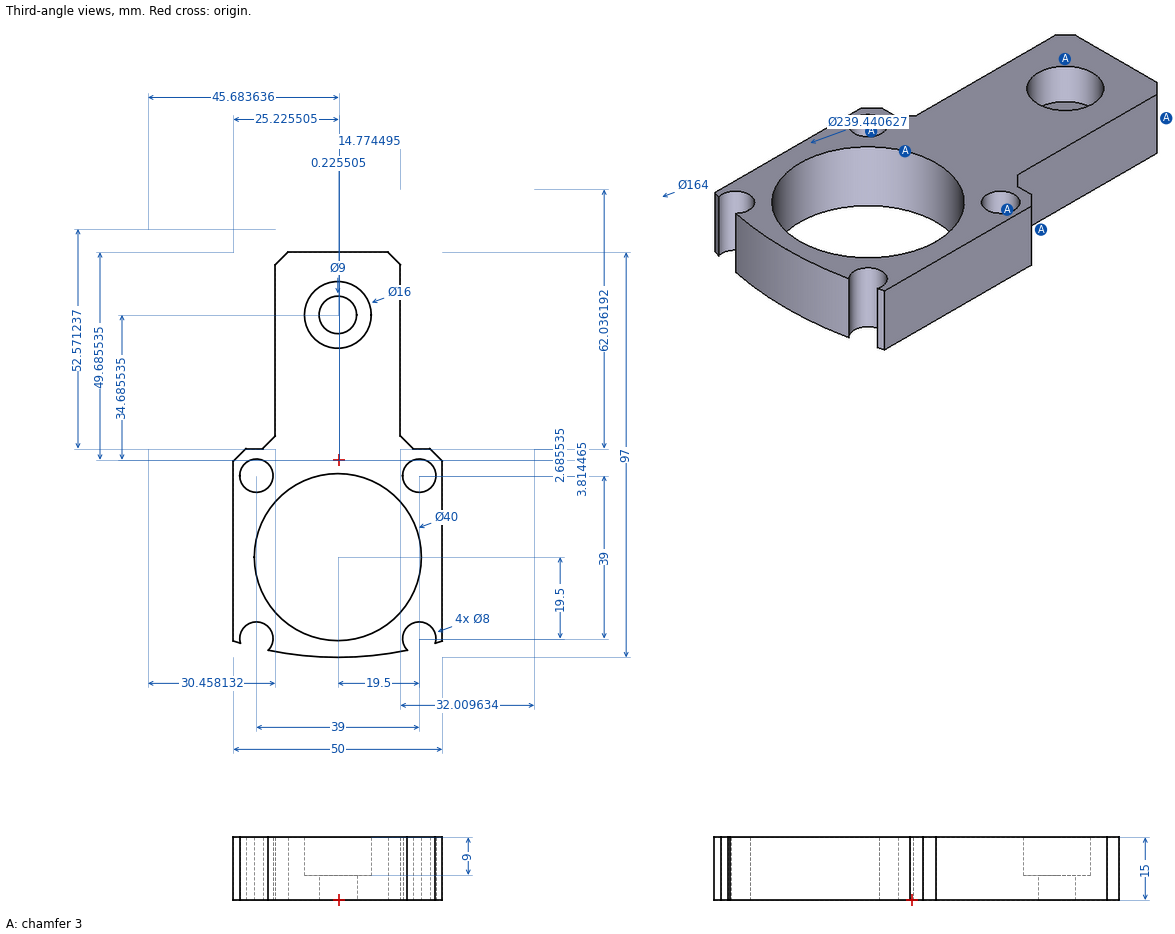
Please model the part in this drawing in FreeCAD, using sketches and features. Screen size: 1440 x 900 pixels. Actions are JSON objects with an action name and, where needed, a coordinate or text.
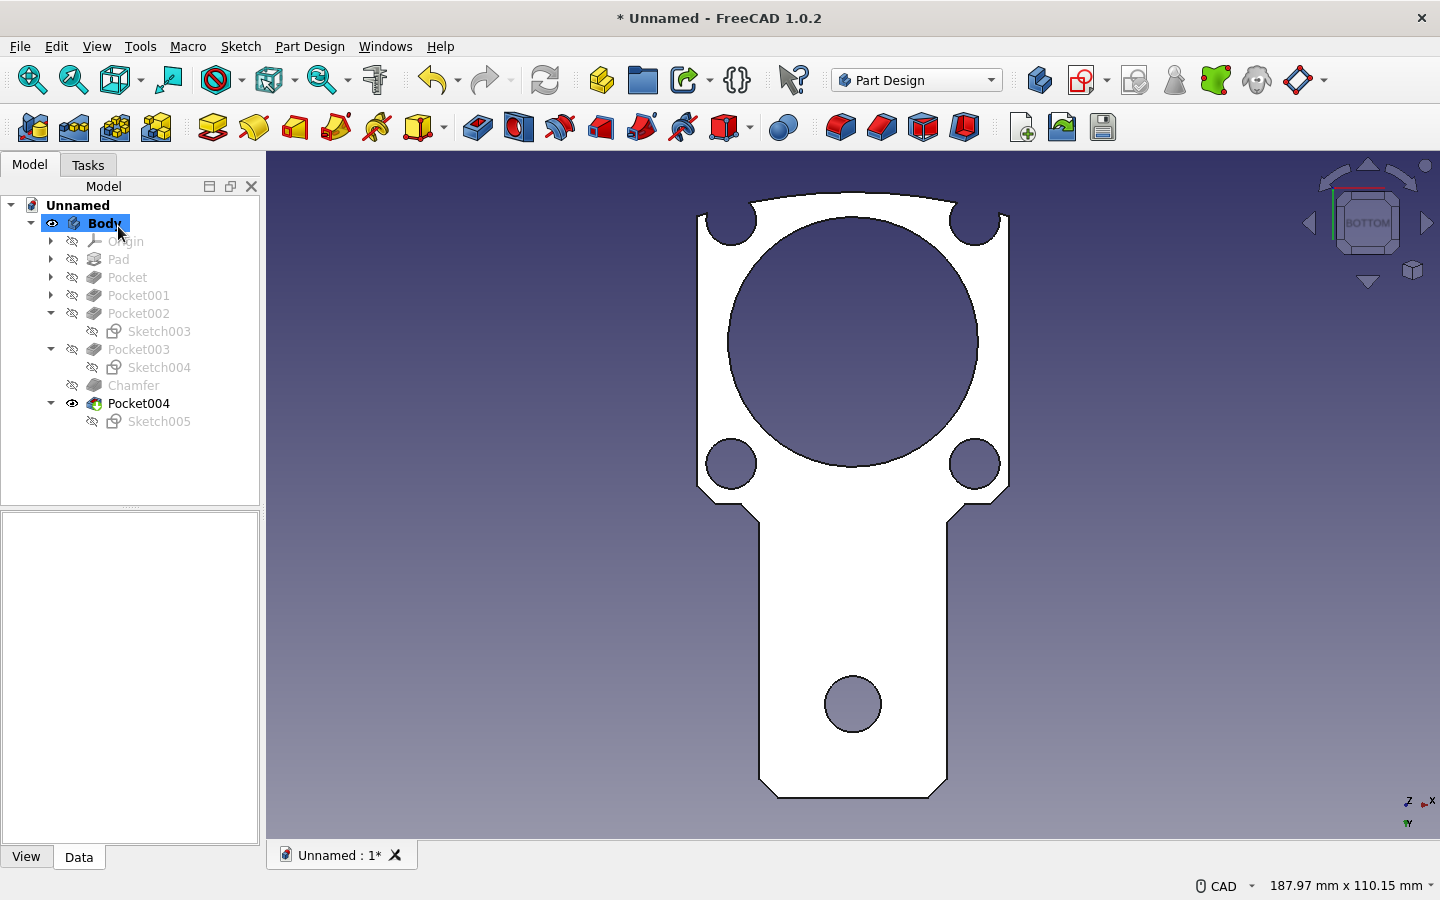
{"action": "key", "text": "0"}